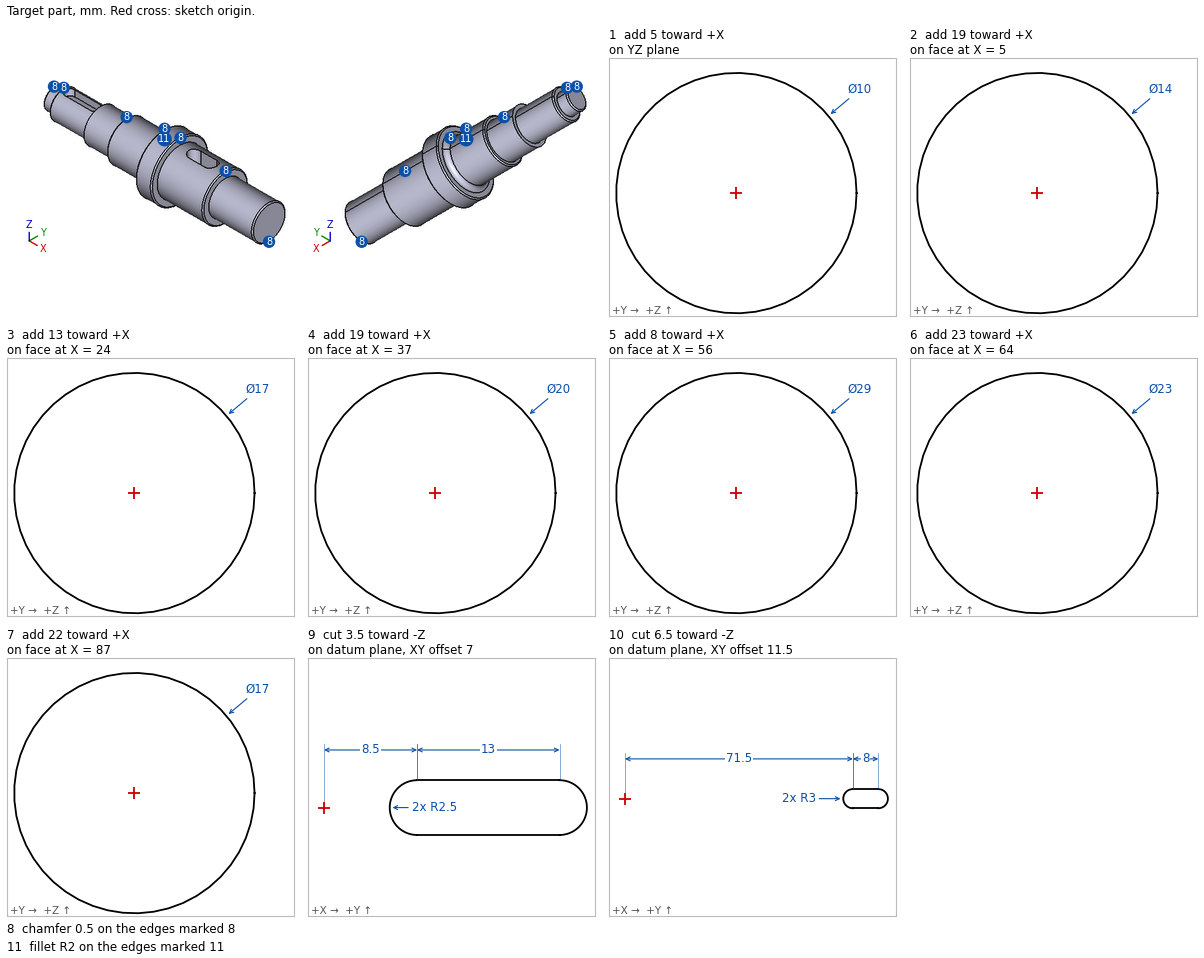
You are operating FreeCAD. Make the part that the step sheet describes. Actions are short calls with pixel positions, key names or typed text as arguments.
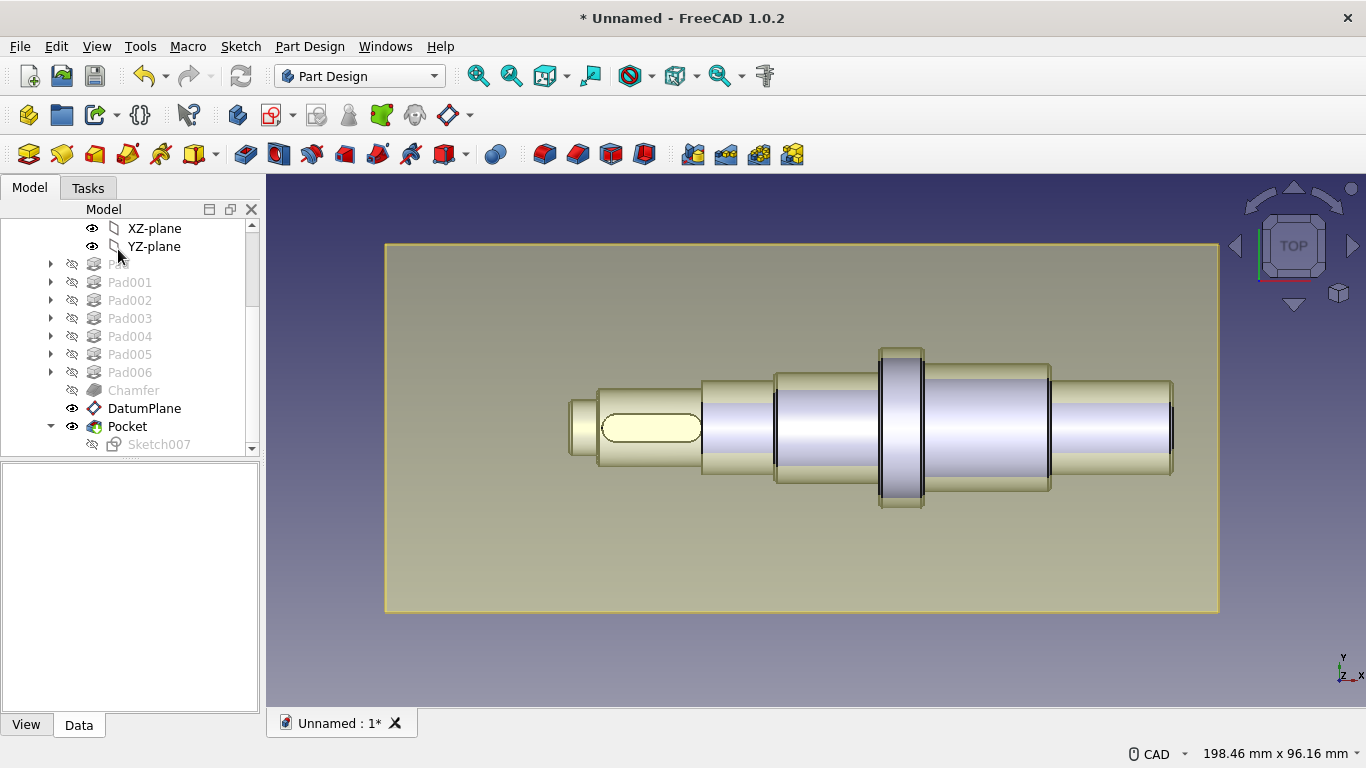
click(117, 408)
key(space)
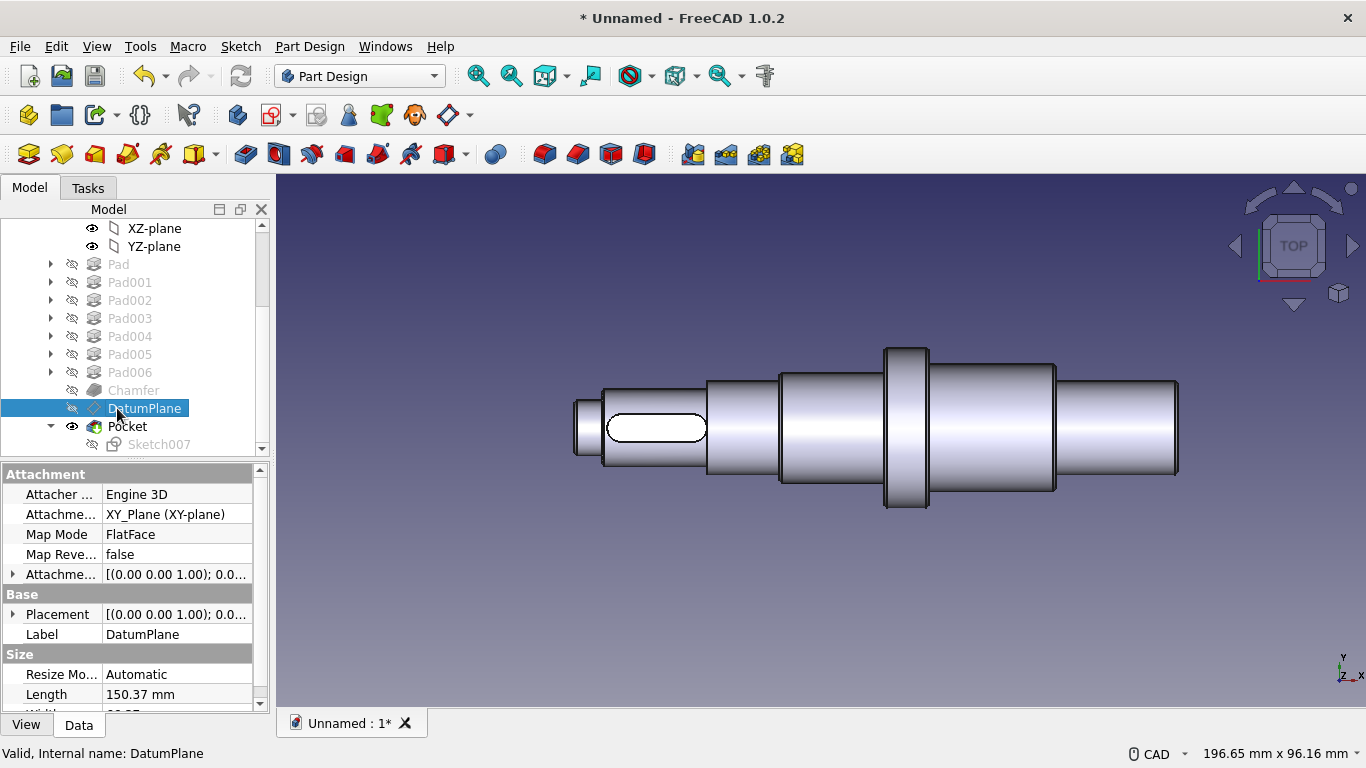
scroll(161, 332, down, 3)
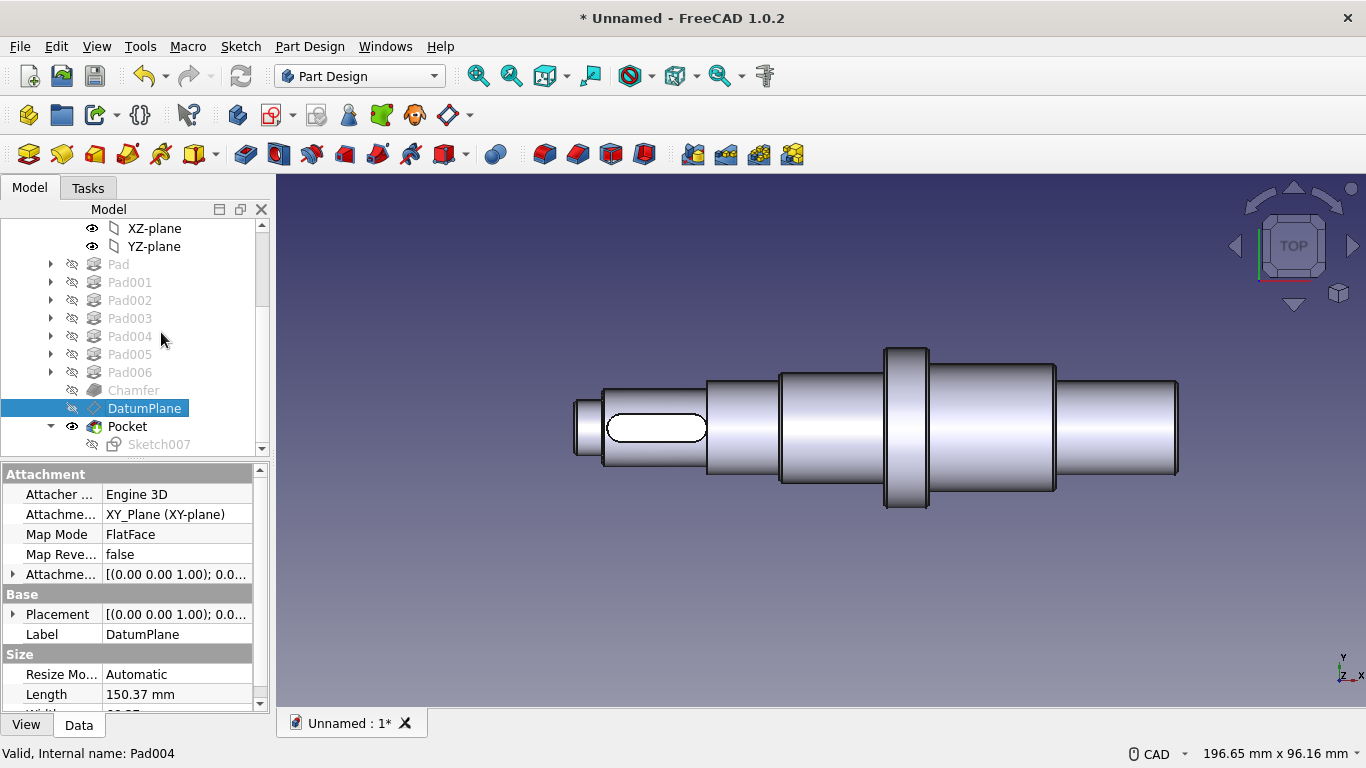
scroll(161, 332, up, 15)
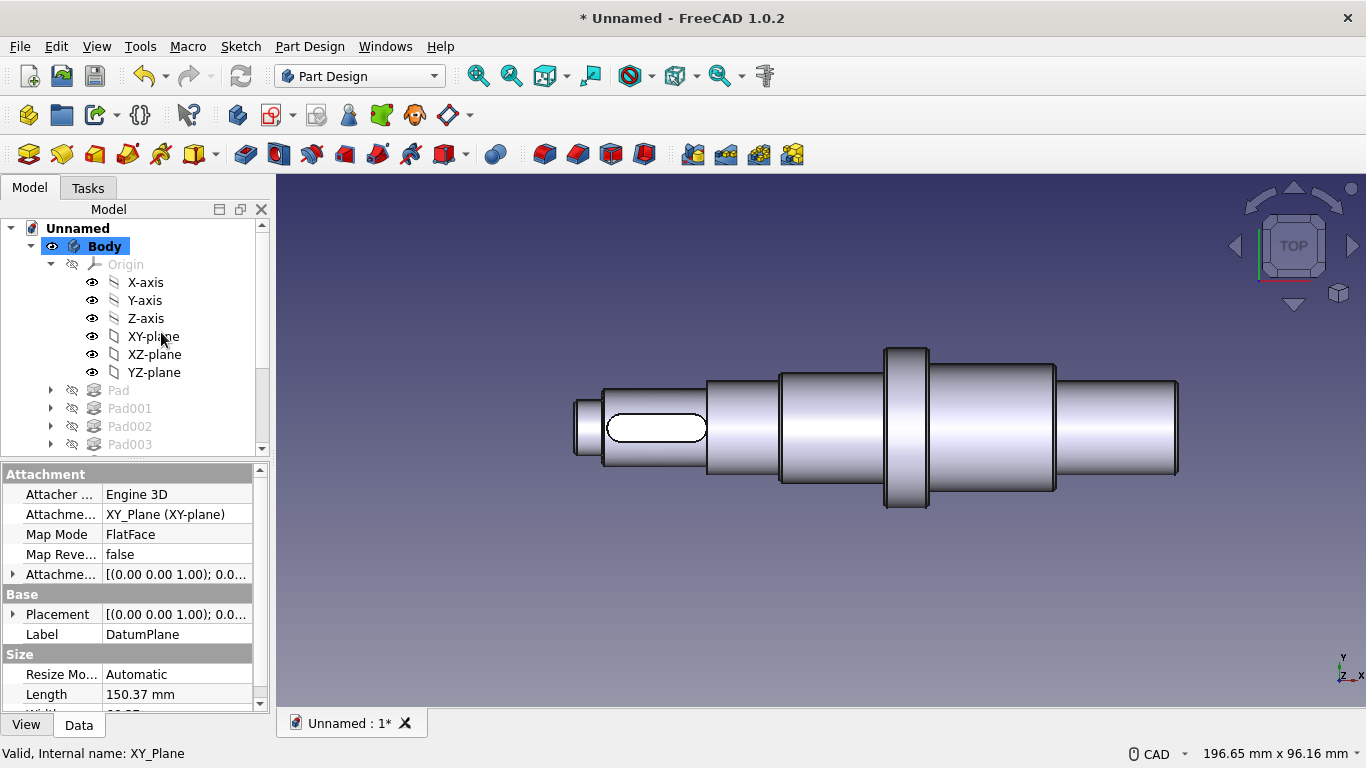
click(137, 336)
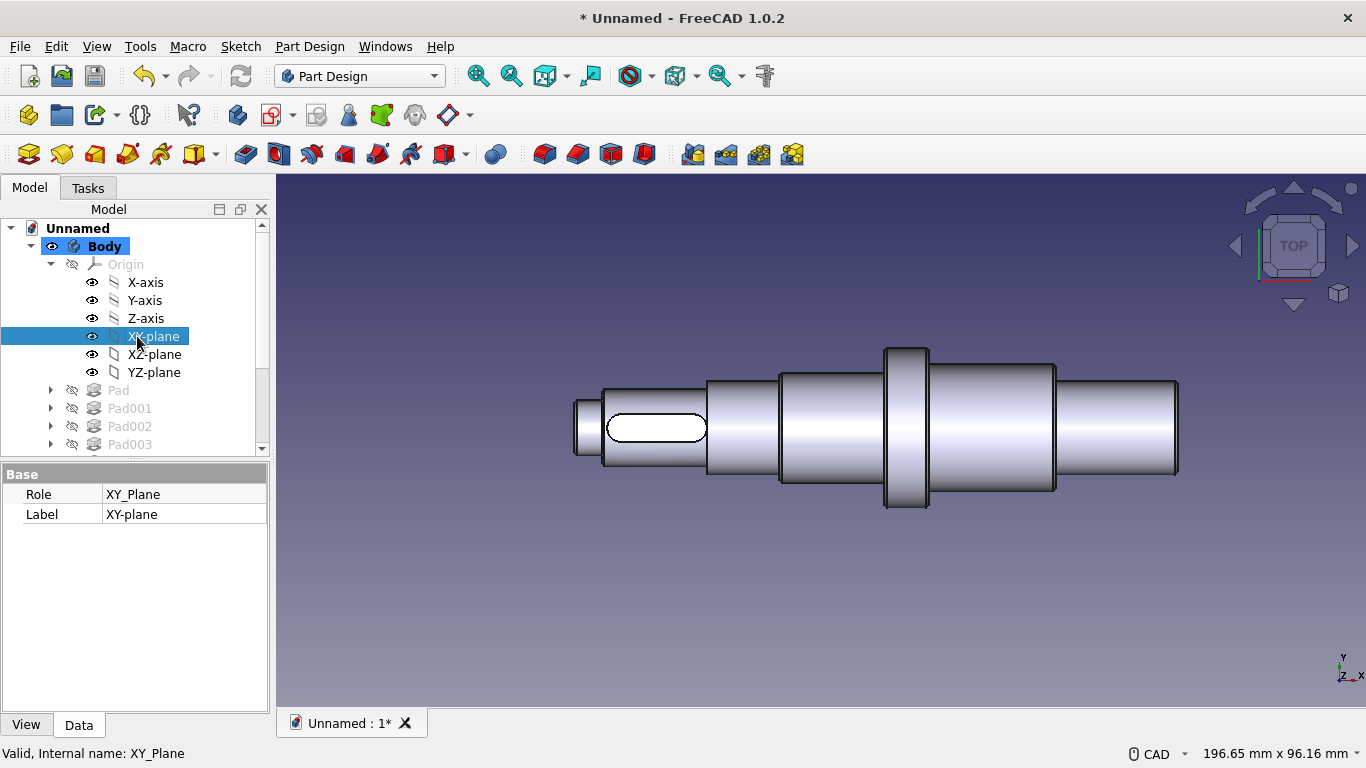
click(448, 116)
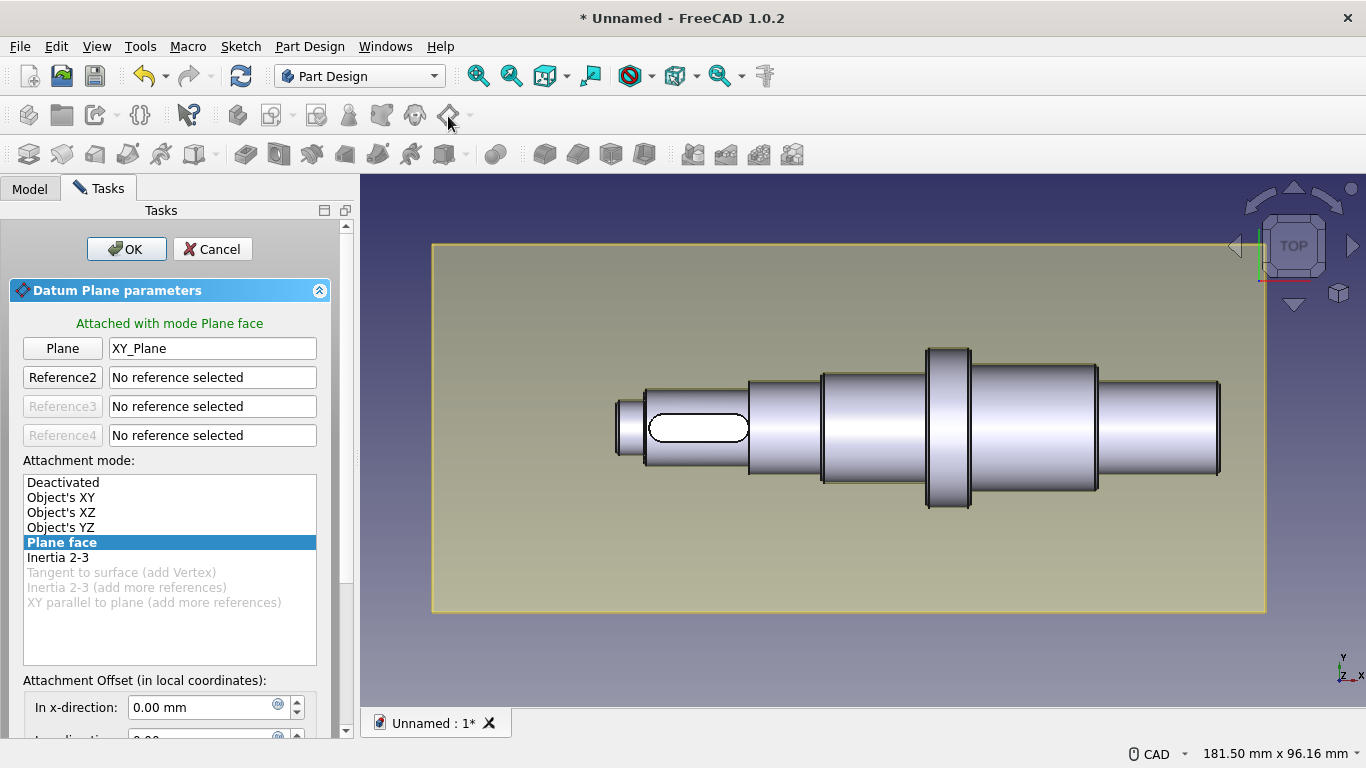
scroll(346, 479, down, 2)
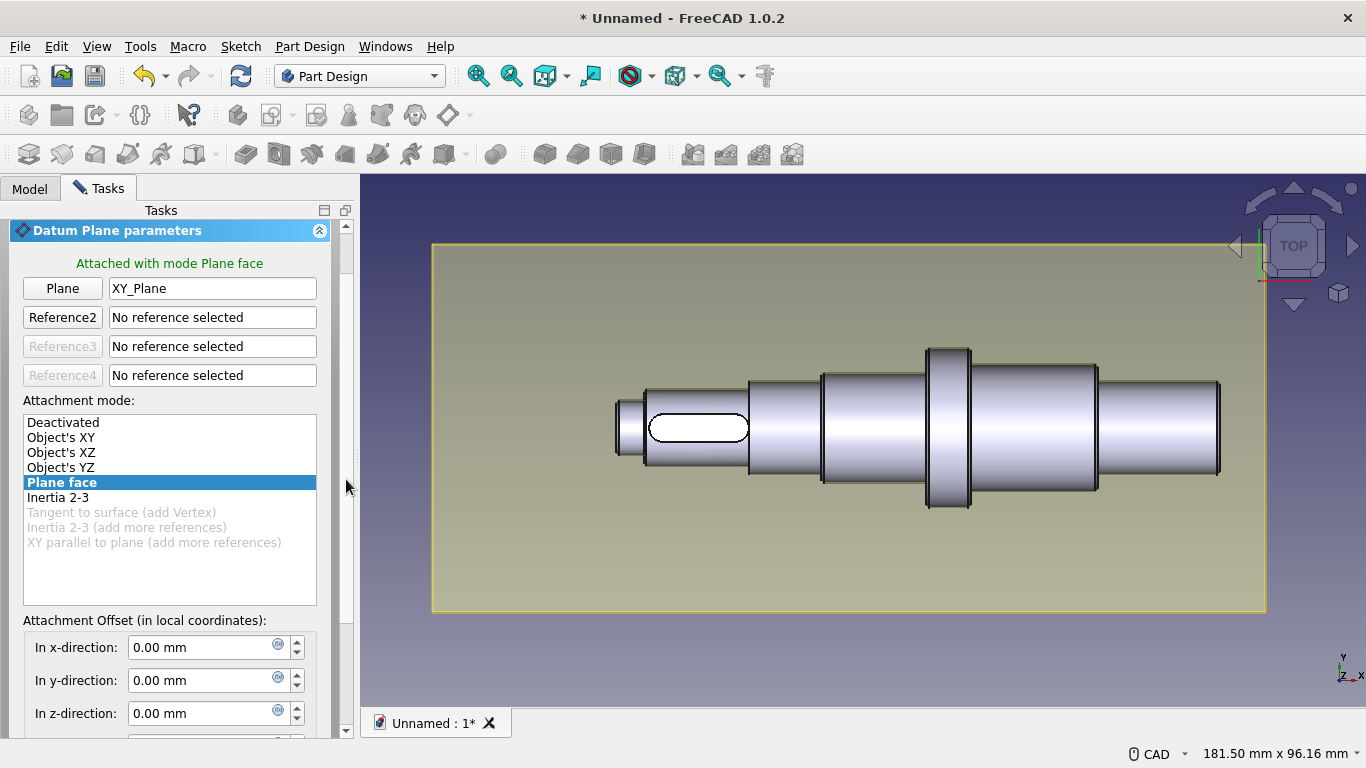
triple_click(210, 654)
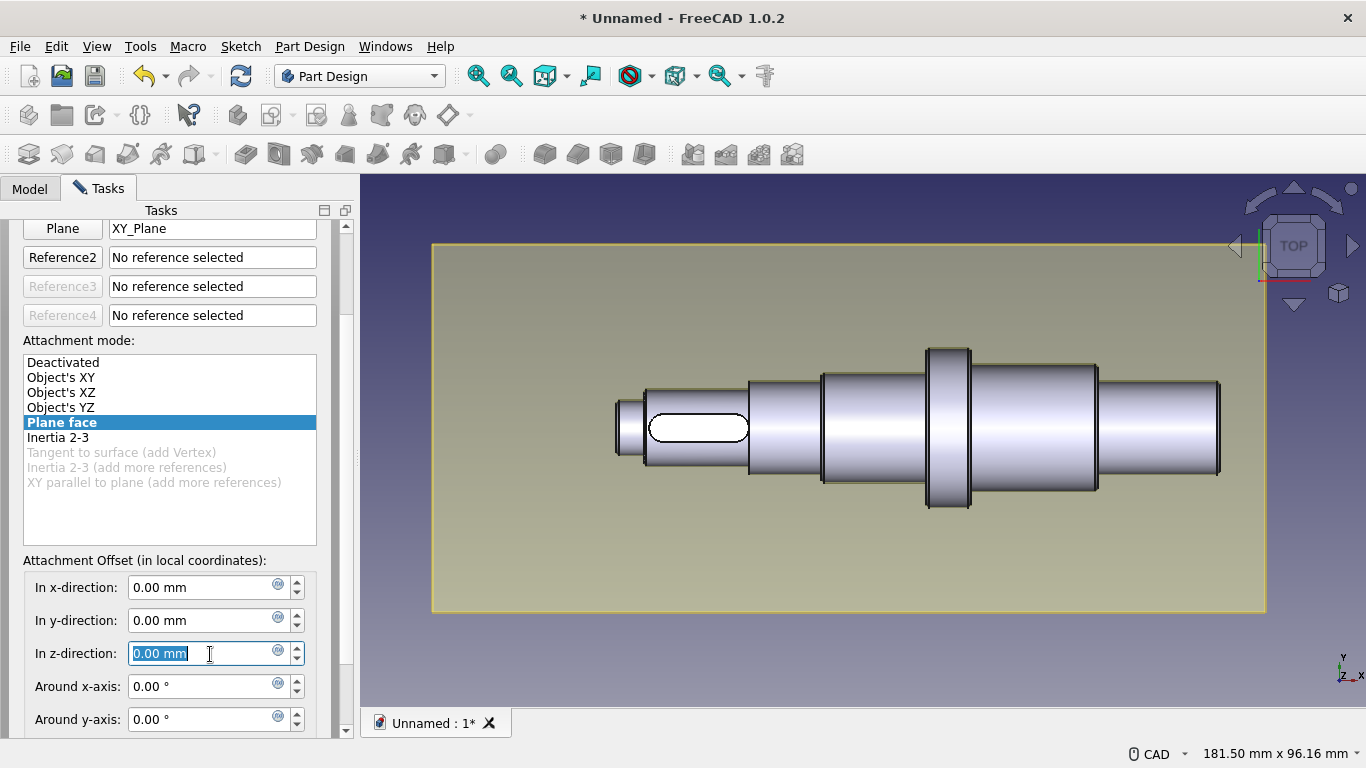
text(11.5)
key(Tab)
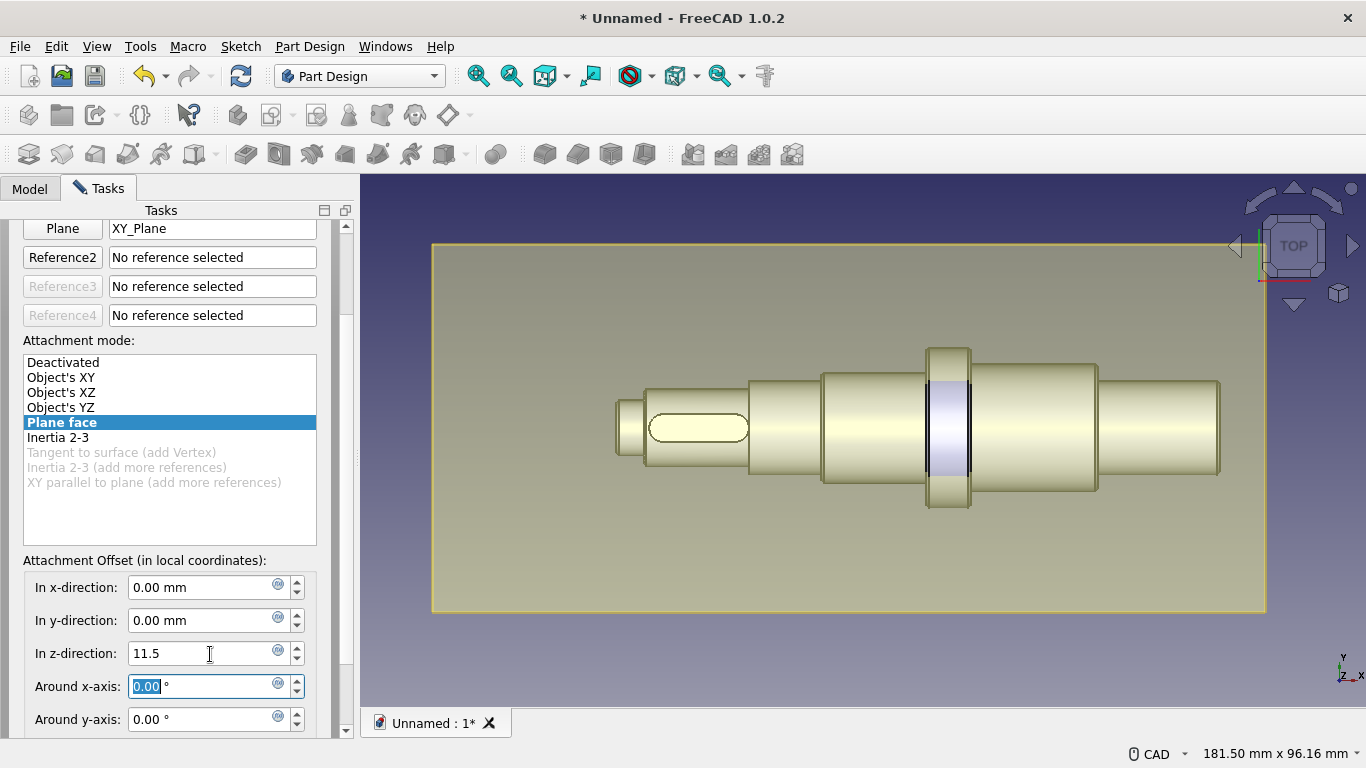
scroll(346, 479, up, 3)